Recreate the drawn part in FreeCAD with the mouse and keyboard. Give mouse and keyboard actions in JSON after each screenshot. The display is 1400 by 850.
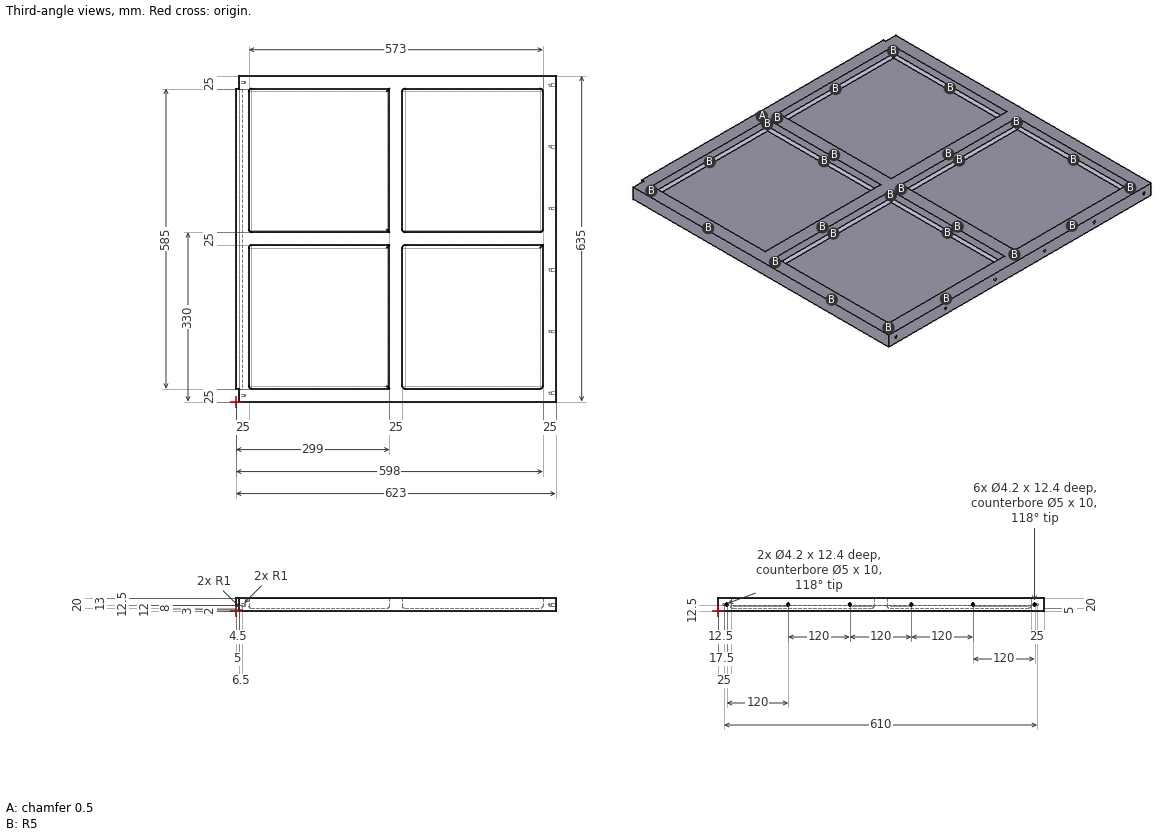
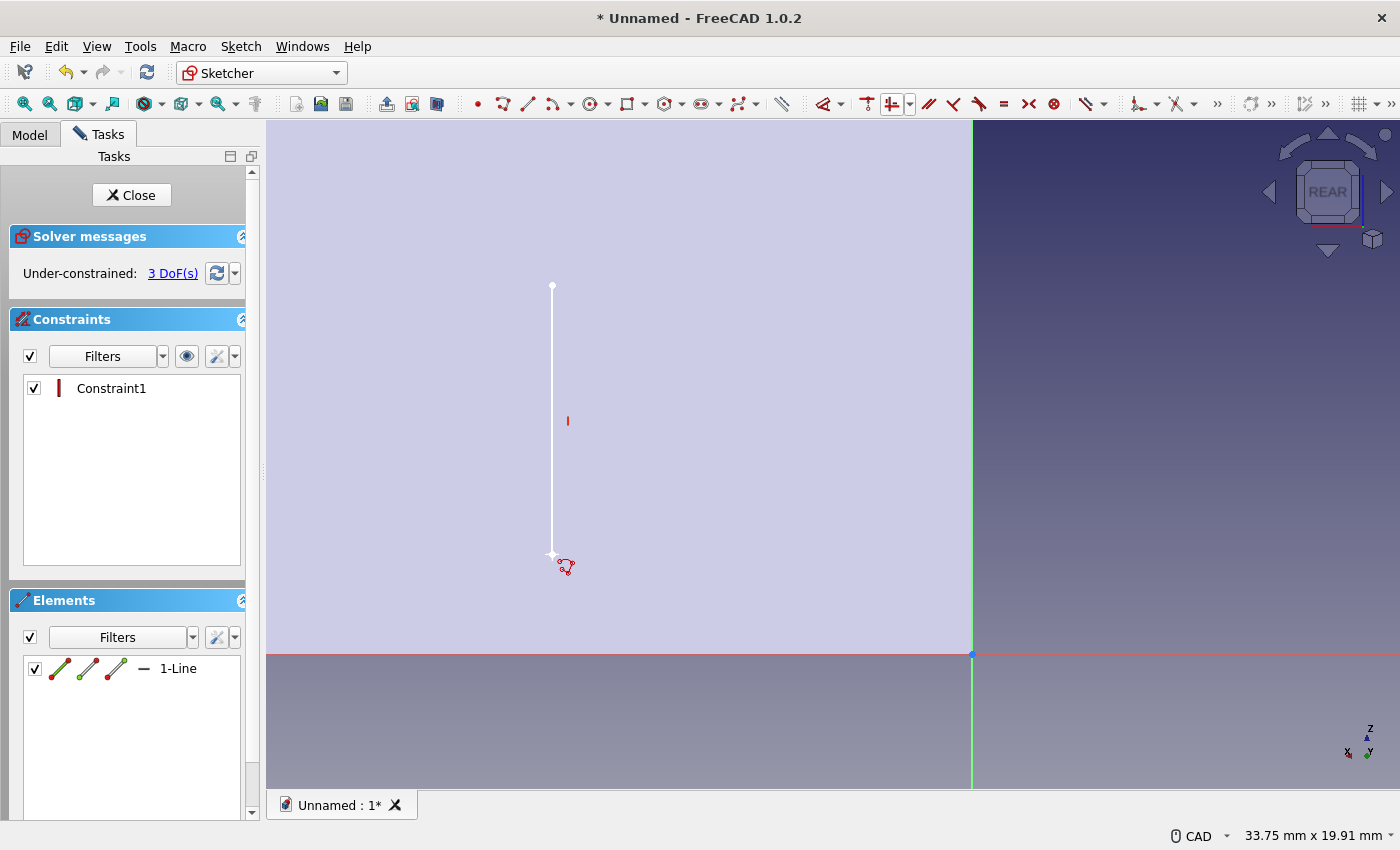
{"action": "left_click", "coordinate": [586, 588]}
{"action": "left_click", "coordinate": [804, 588]}
{"action": "left_click", "coordinate": [804, 655]}
{"action": "left_click", "coordinate": [972, 655]}
{"action": "left_click", "coordinate": [963, 251]}
{"action": "left_click", "coordinate": [586, 251]}
{"action": "right_click", "coordinate": [586, 251]}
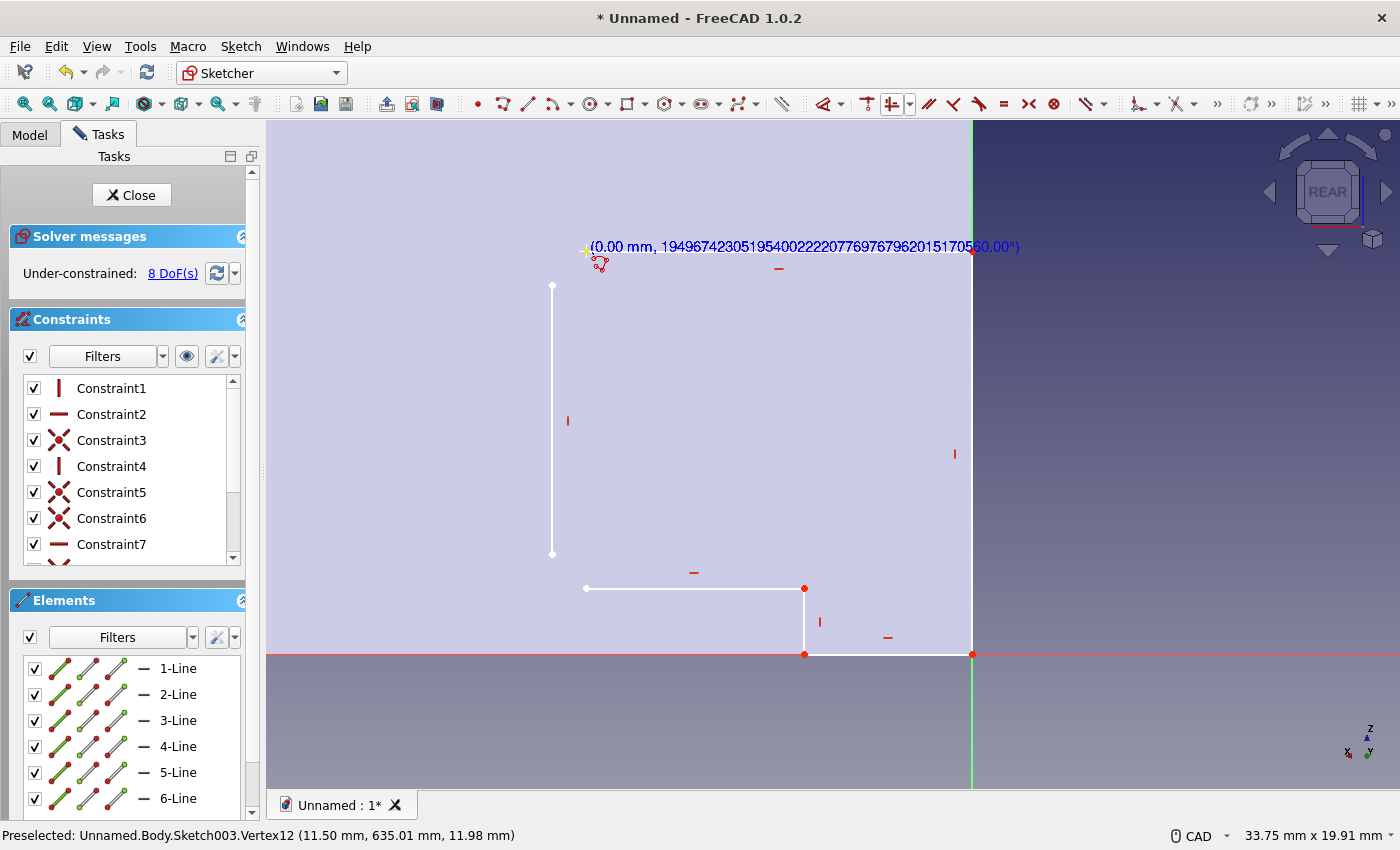
{"action": "key", "text": "g 3 a"}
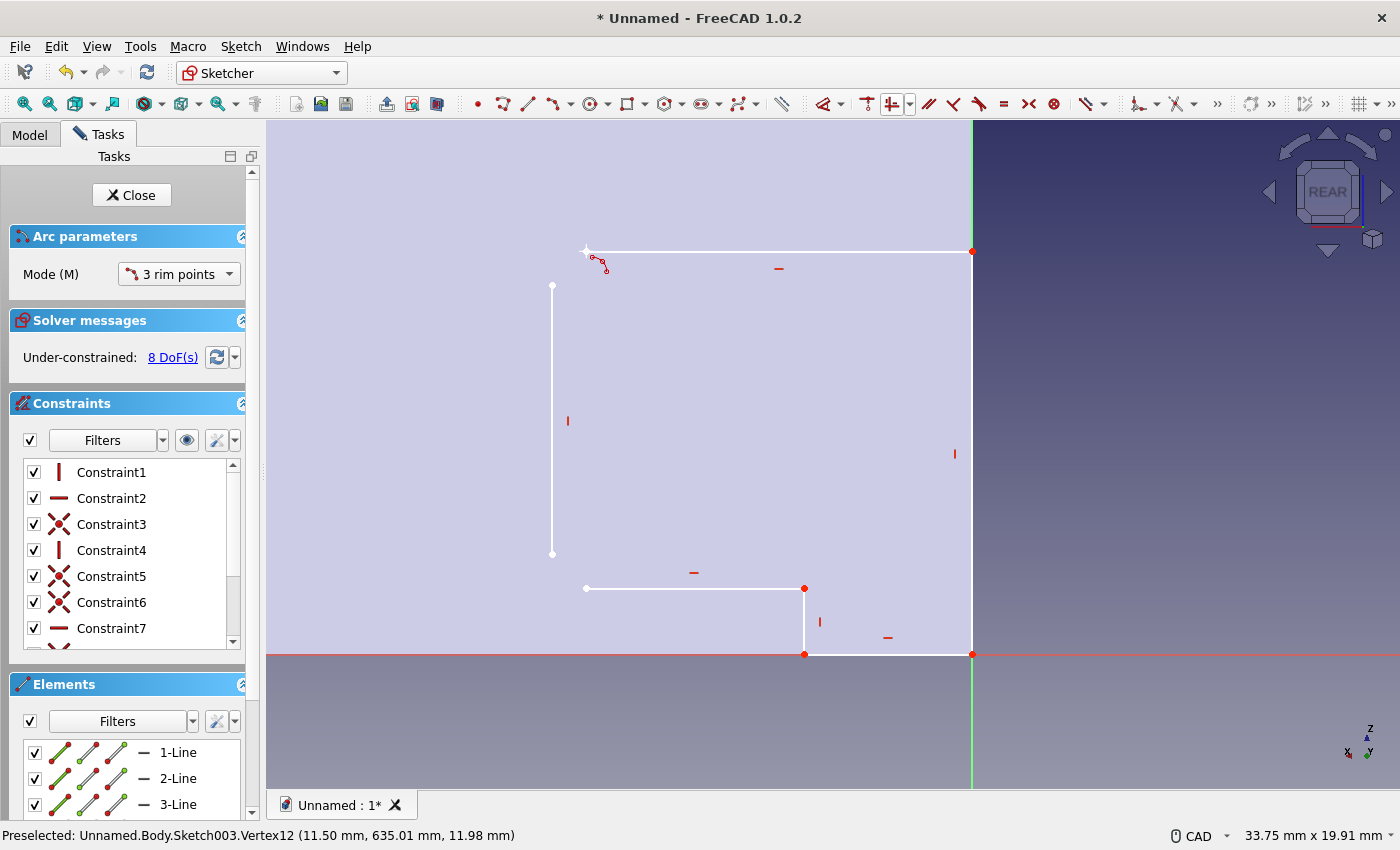
{"action": "left_click", "coordinate": [552, 555]}
{"action": "left_click", "coordinate": [586, 589]}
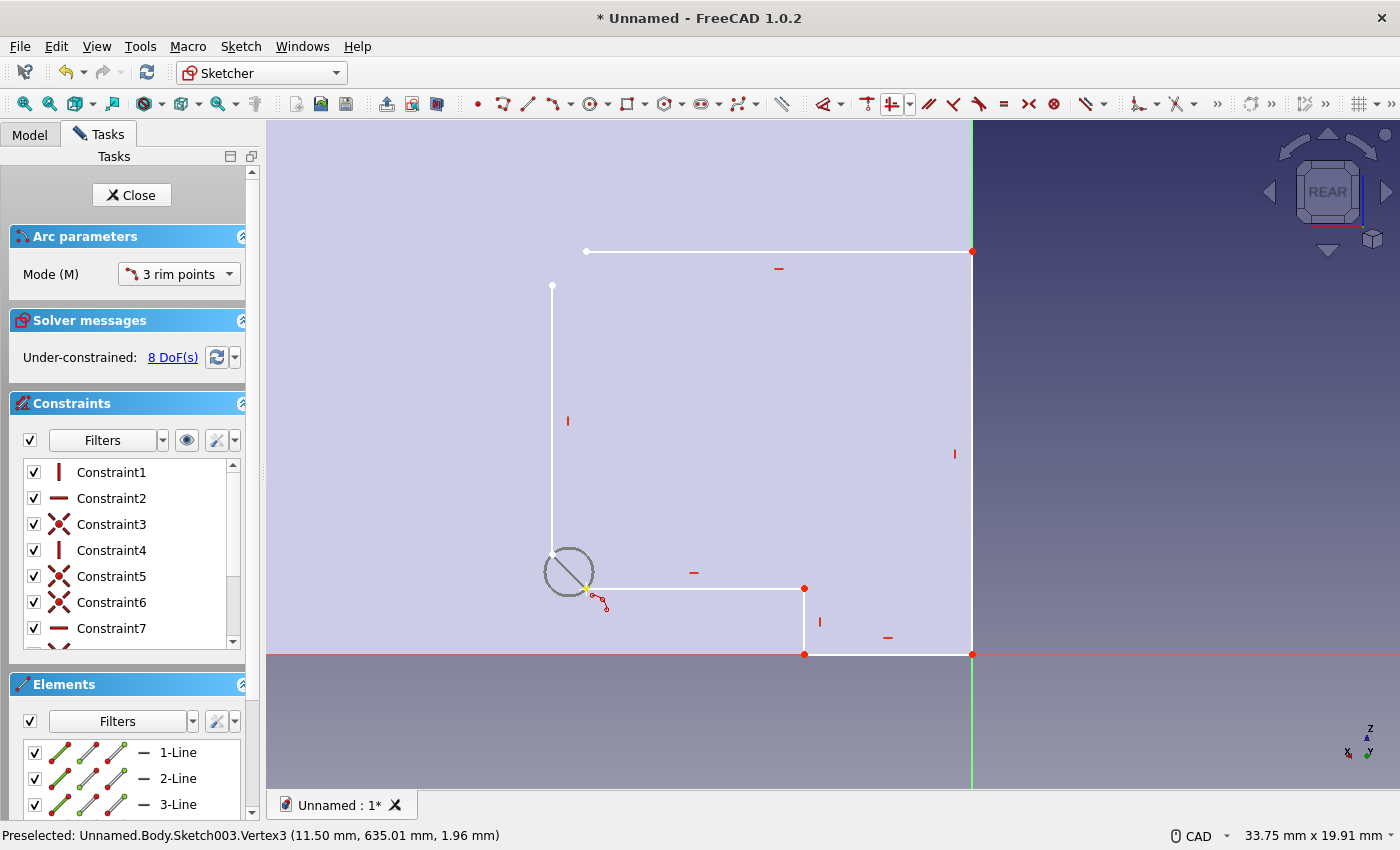
{"action": "scroll", "coordinate": [562, 578], "scroll_direction": "up", "scroll_amount": 3}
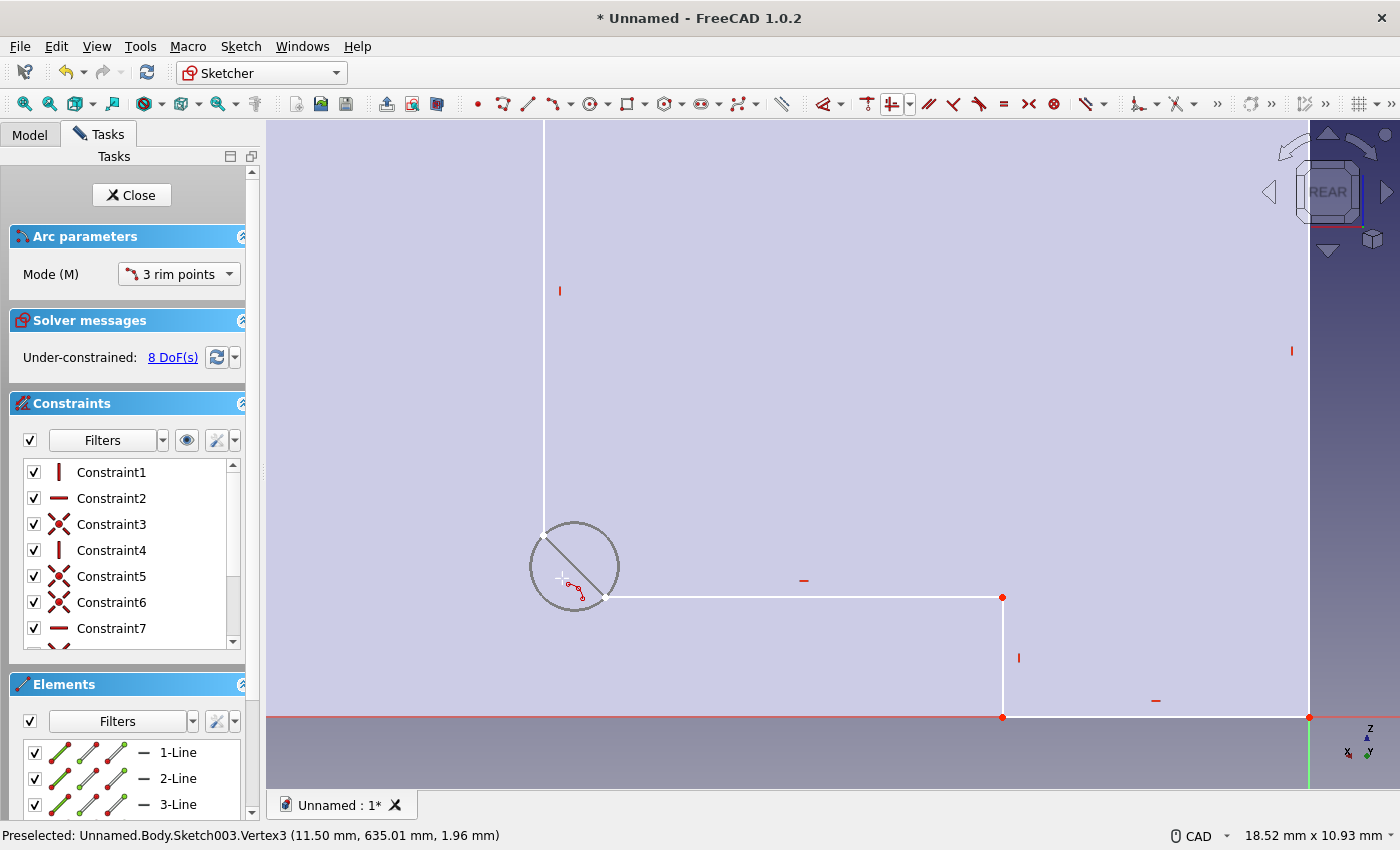
{"action": "left_click", "coordinate": [562, 577]}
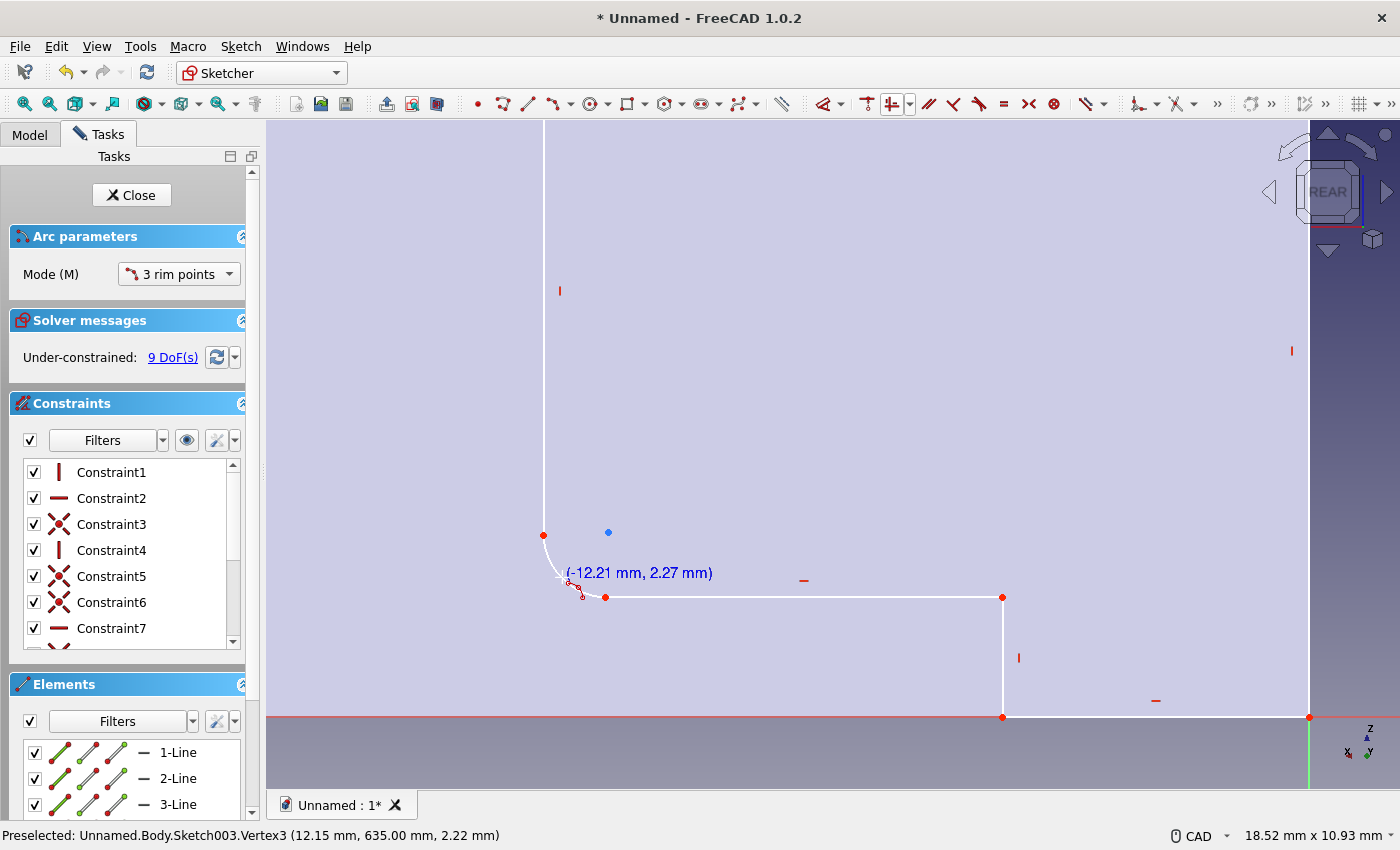
{"action": "scroll", "coordinate": [567, 582], "scroll_direction": "down", "scroll_amount": 3}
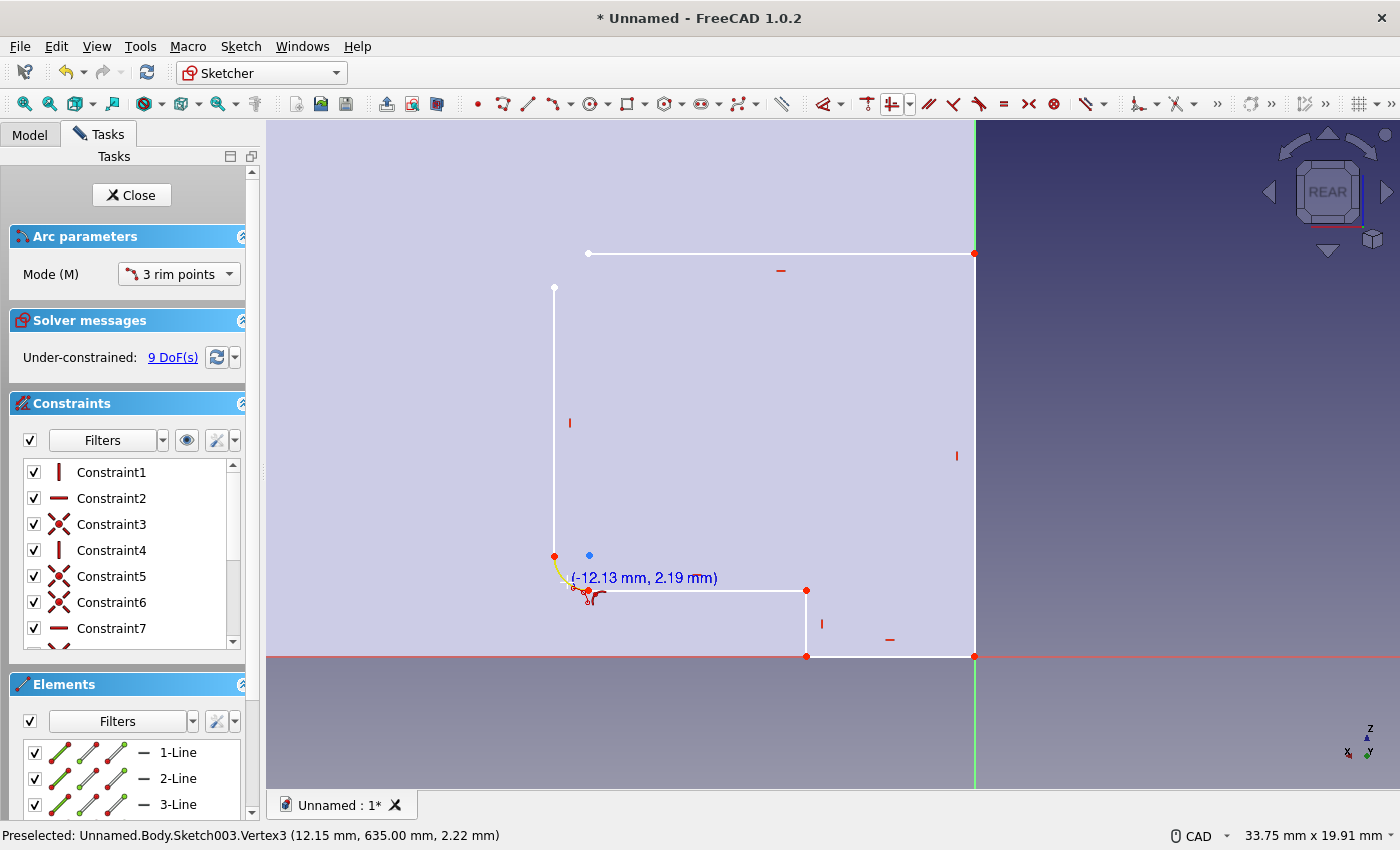
{"action": "left_click", "coordinate": [588, 254]}
{"action": "left_click", "coordinate": [554, 288]}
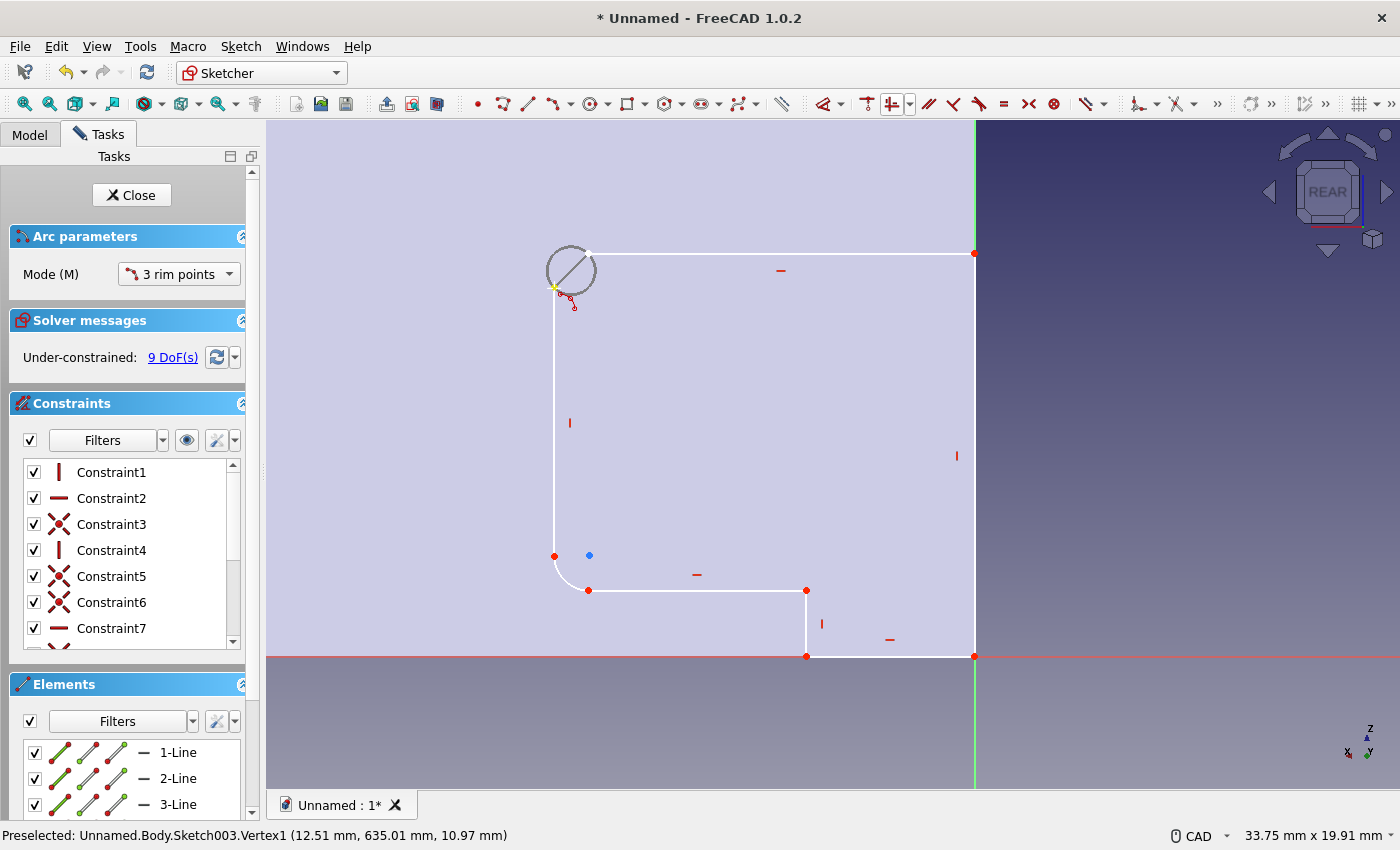
{"action": "scroll", "coordinate": [564, 263], "scroll_direction": "up", "scroll_amount": 3}